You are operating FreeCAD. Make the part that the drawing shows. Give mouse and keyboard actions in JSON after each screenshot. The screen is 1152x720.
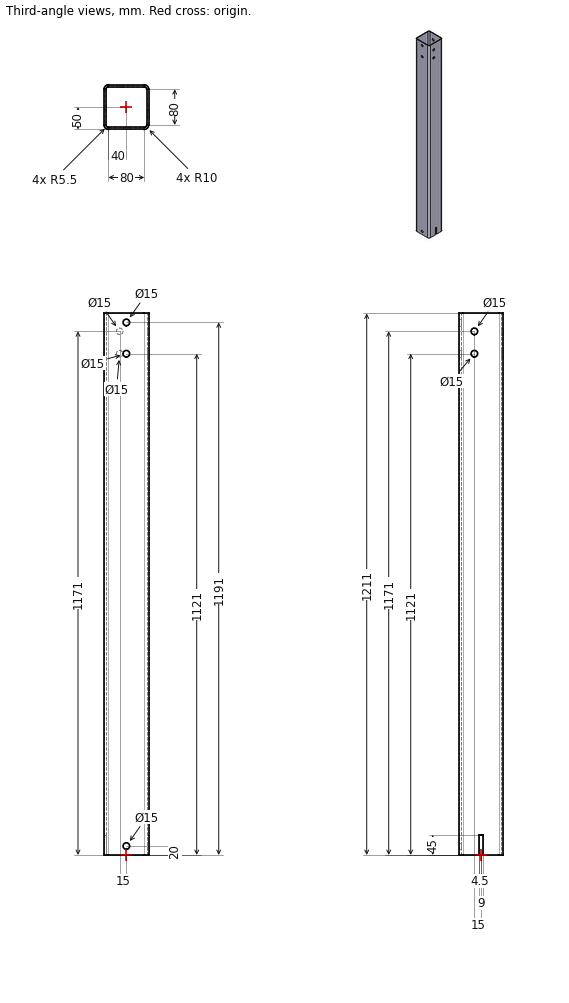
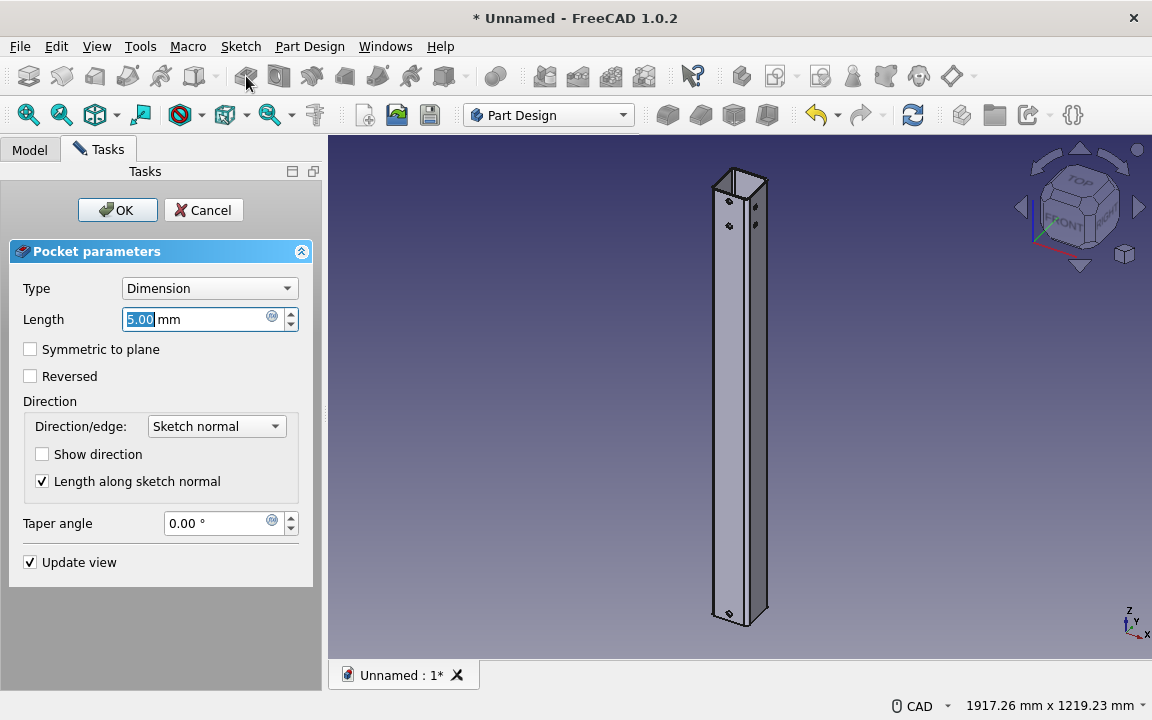
{"action": "left_click", "coordinate": [210, 288]}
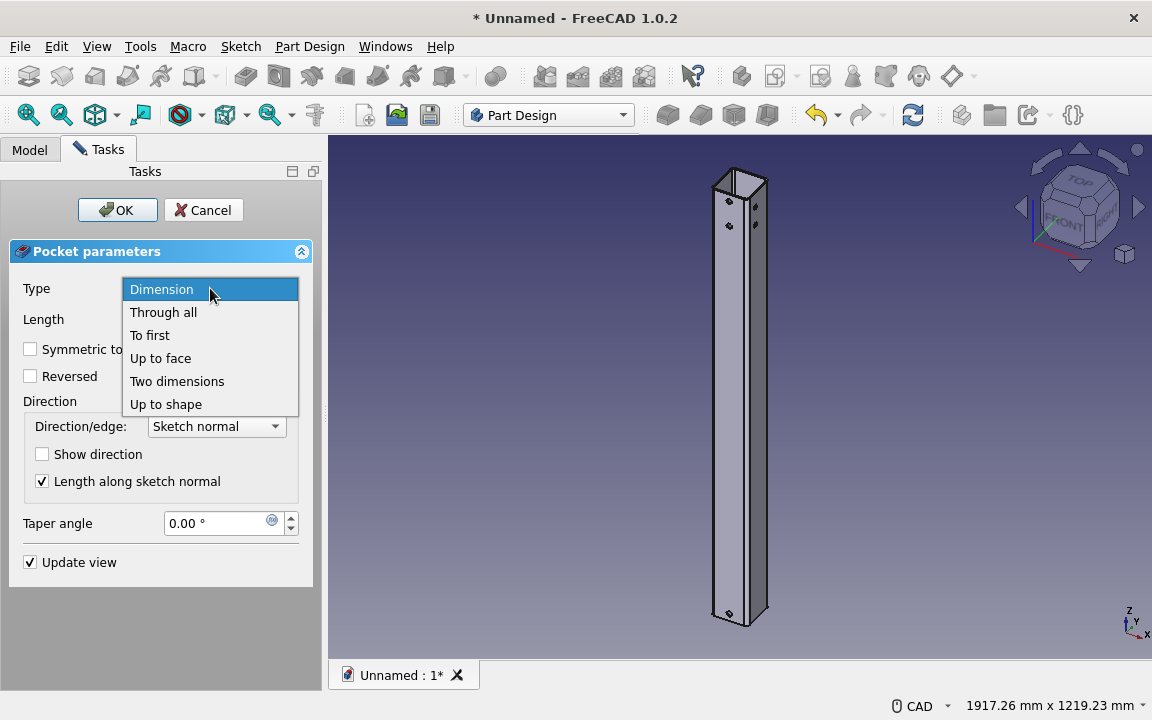
{"action": "left_click", "coordinate": [208, 336]}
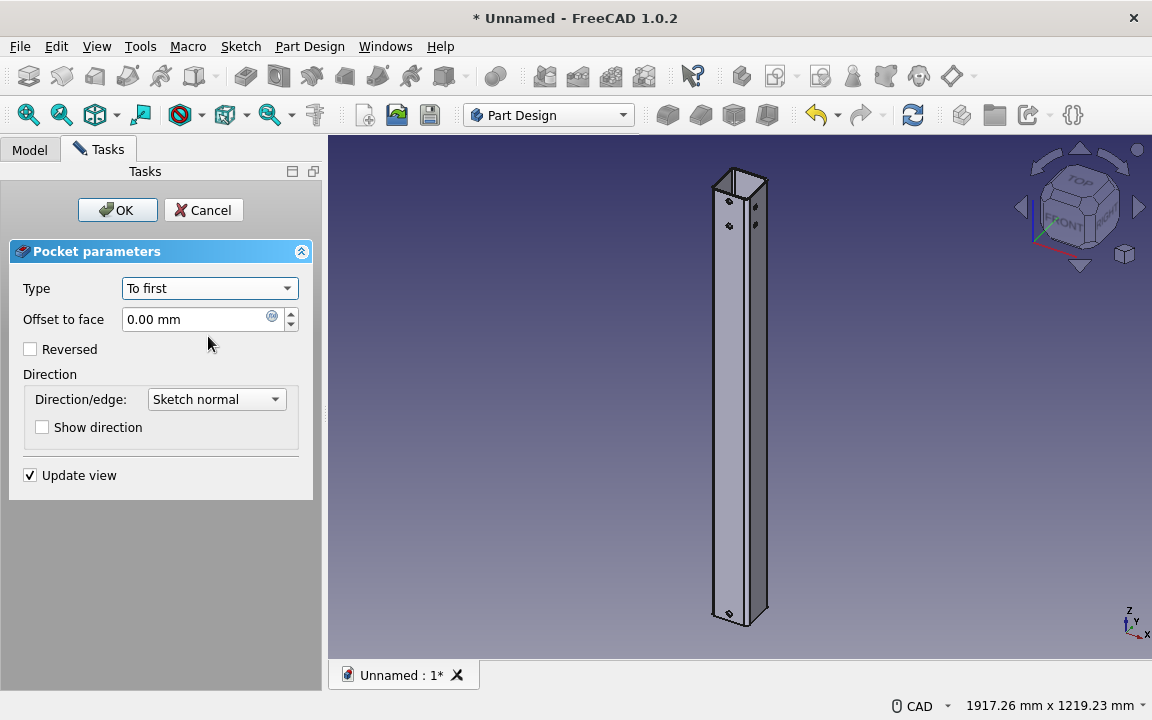
{"action": "left_click", "coordinate": [118, 210]}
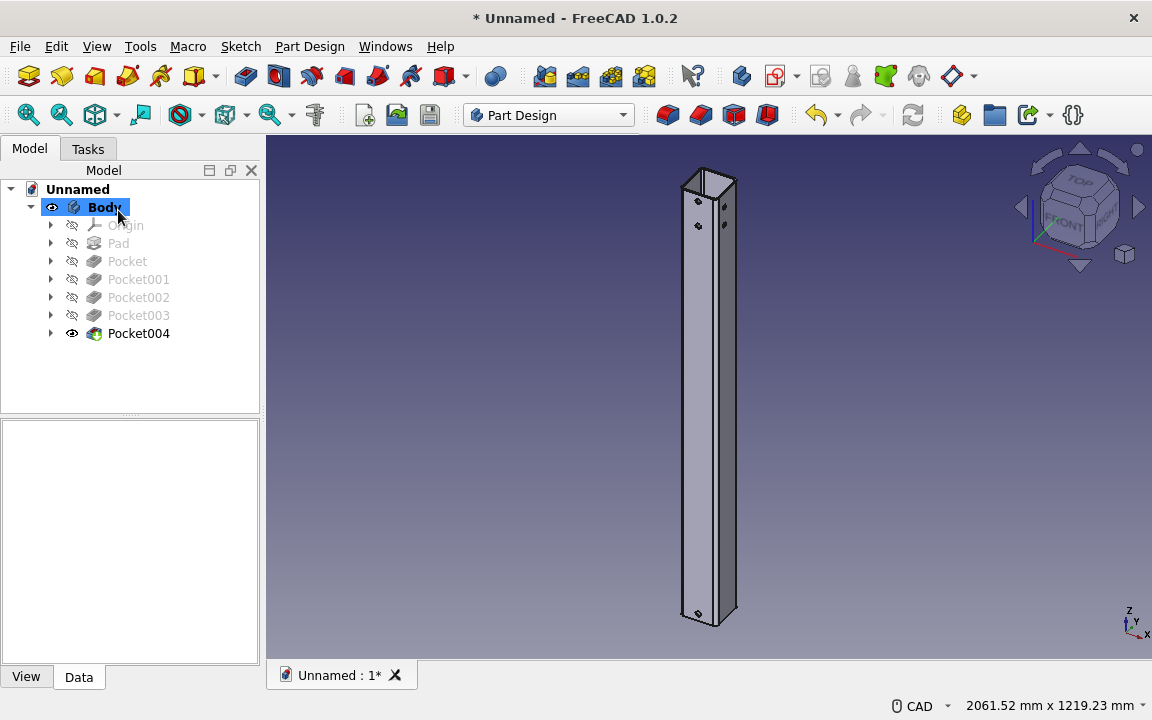
{"action": "key", "text": "4"}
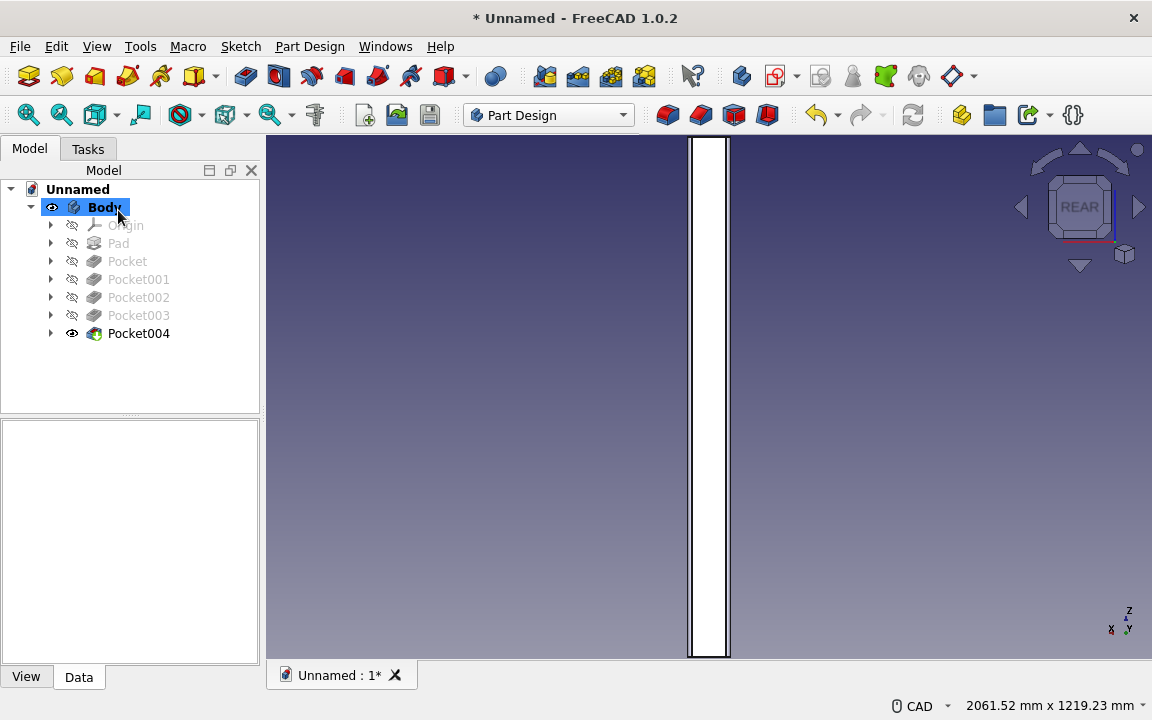
{"action": "left_click", "coordinate": [709, 173]}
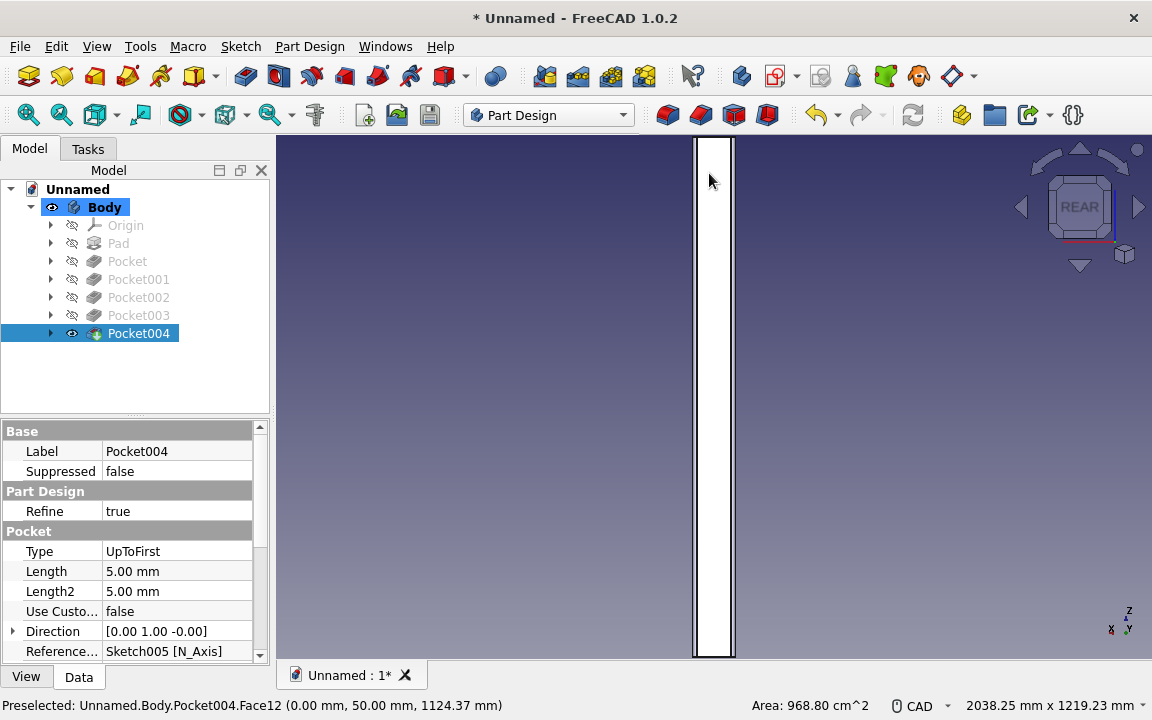
{"action": "left_click", "coordinate": [774, 76]}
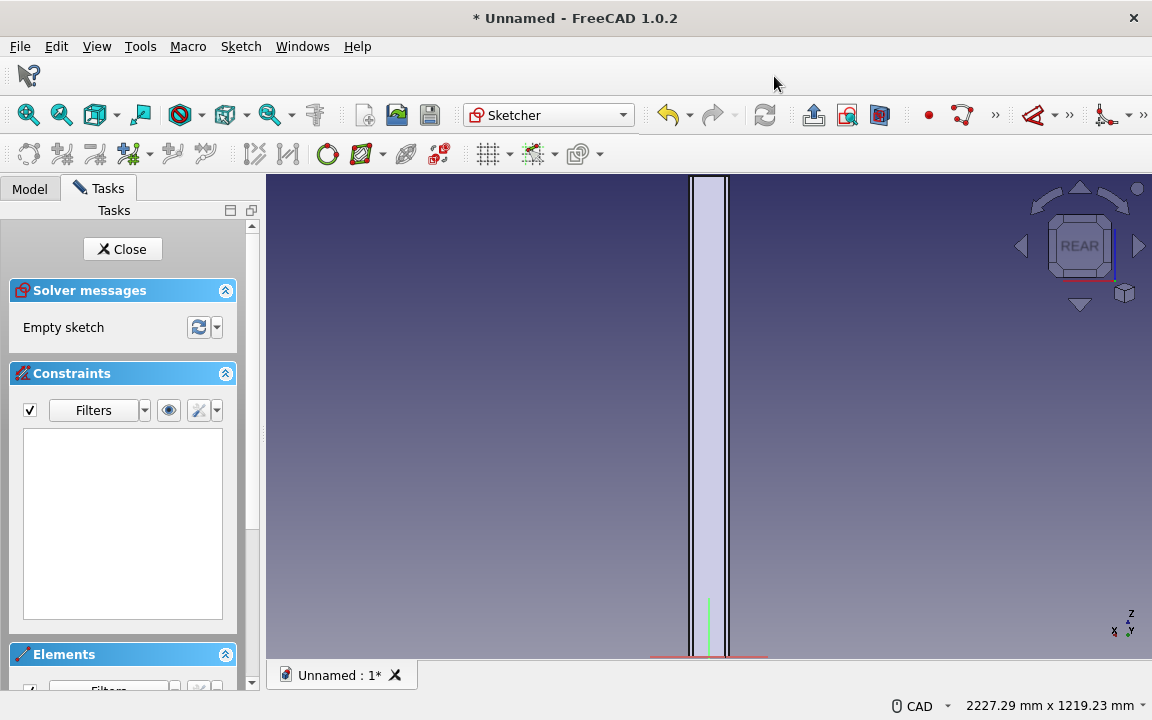
{"action": "scroll", "coordinate": [640, 416], "scroll_direction": "down", "scroll_amount": 5}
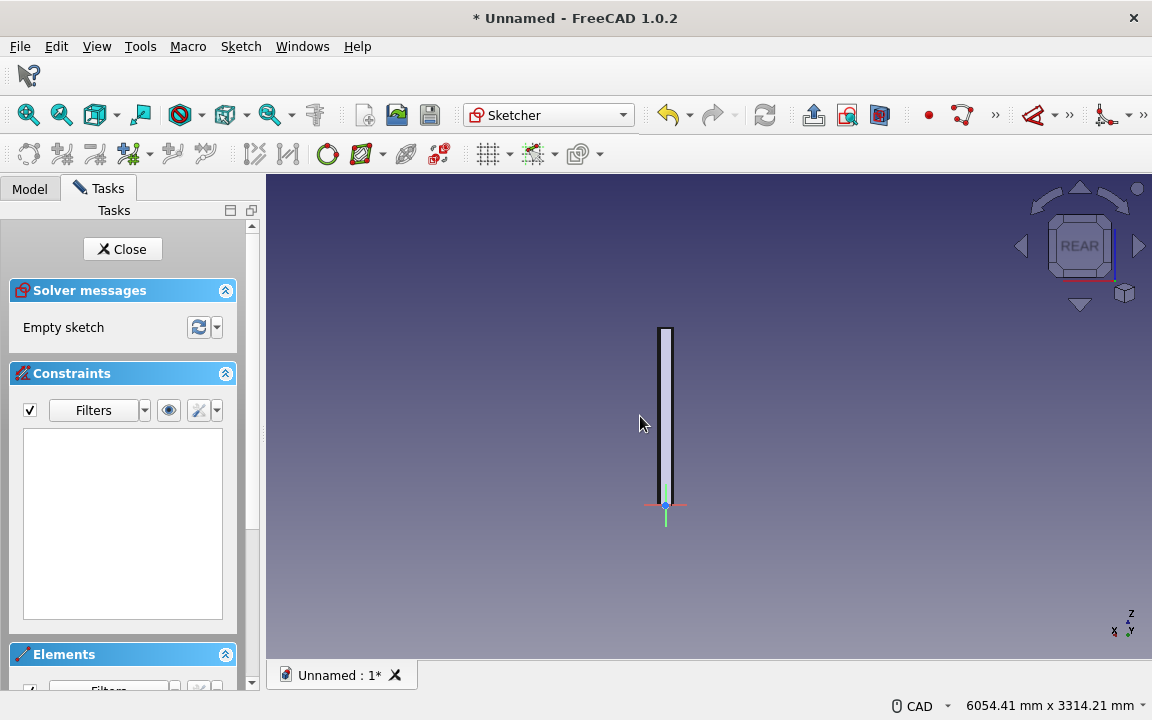
{"action": "scroll", "coordinate": [669, 329], "scroll_direction": "up", "scroll_amount": 15}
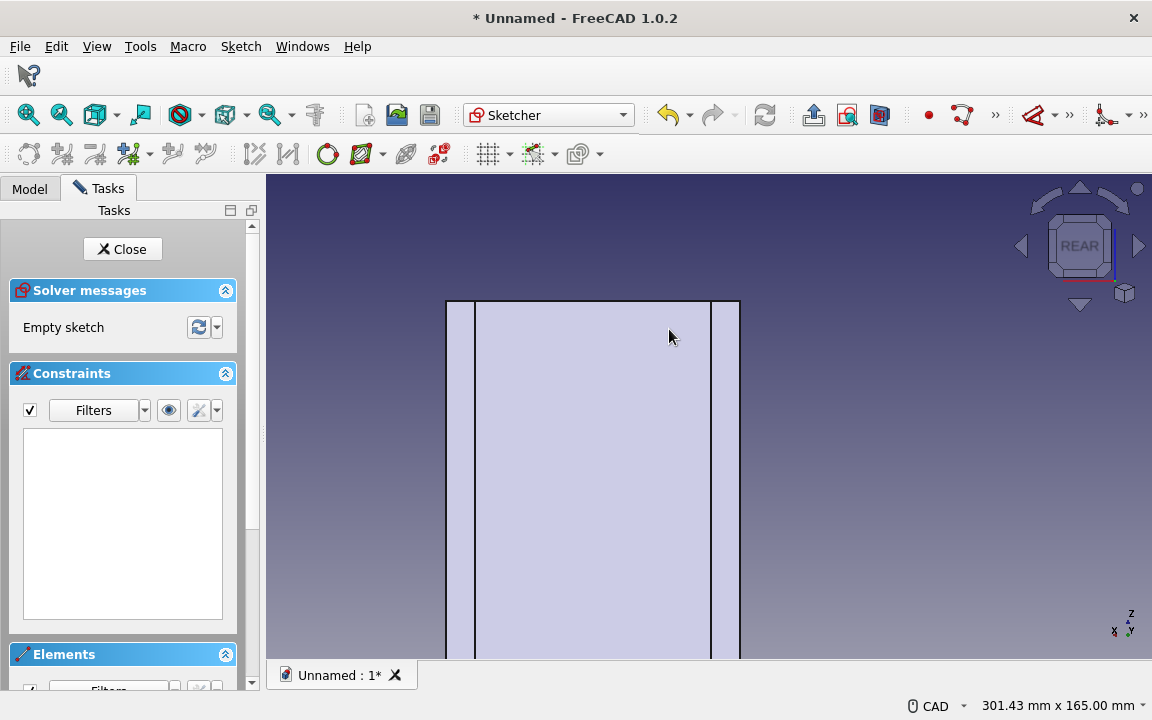
{"action": "scroll", "coordinate": [637, 418], "scroll_direction": "up", "scroll_amount": 10}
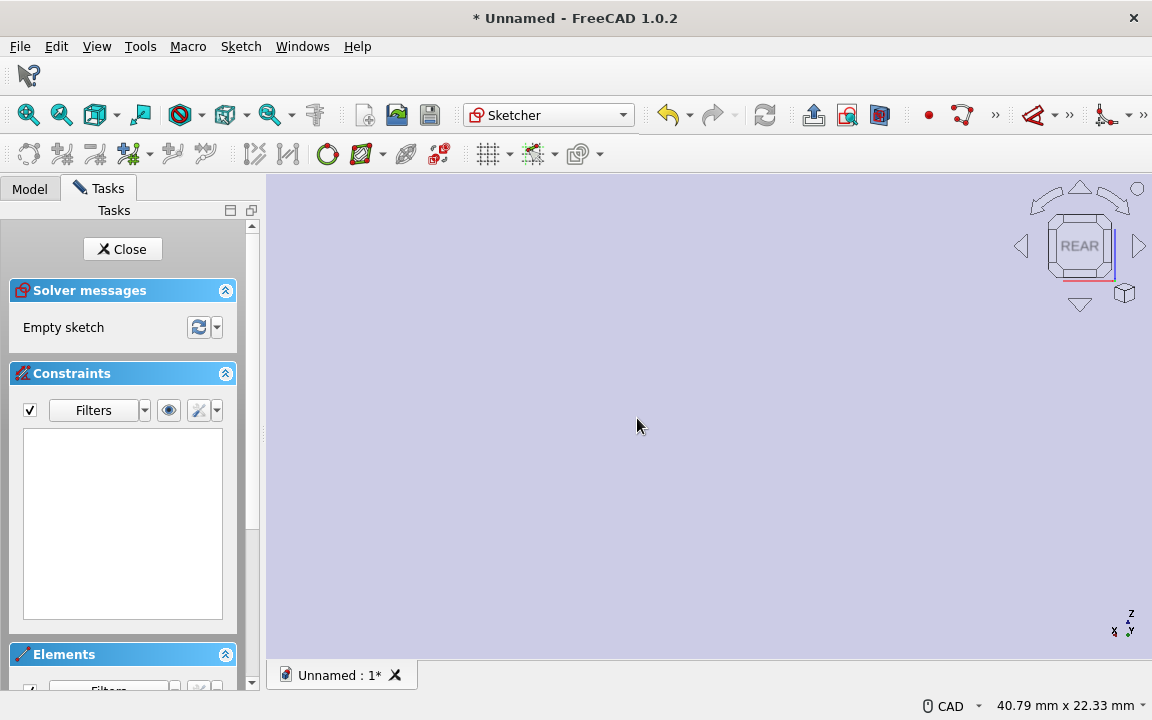
{"action": "key", "text": "g c"}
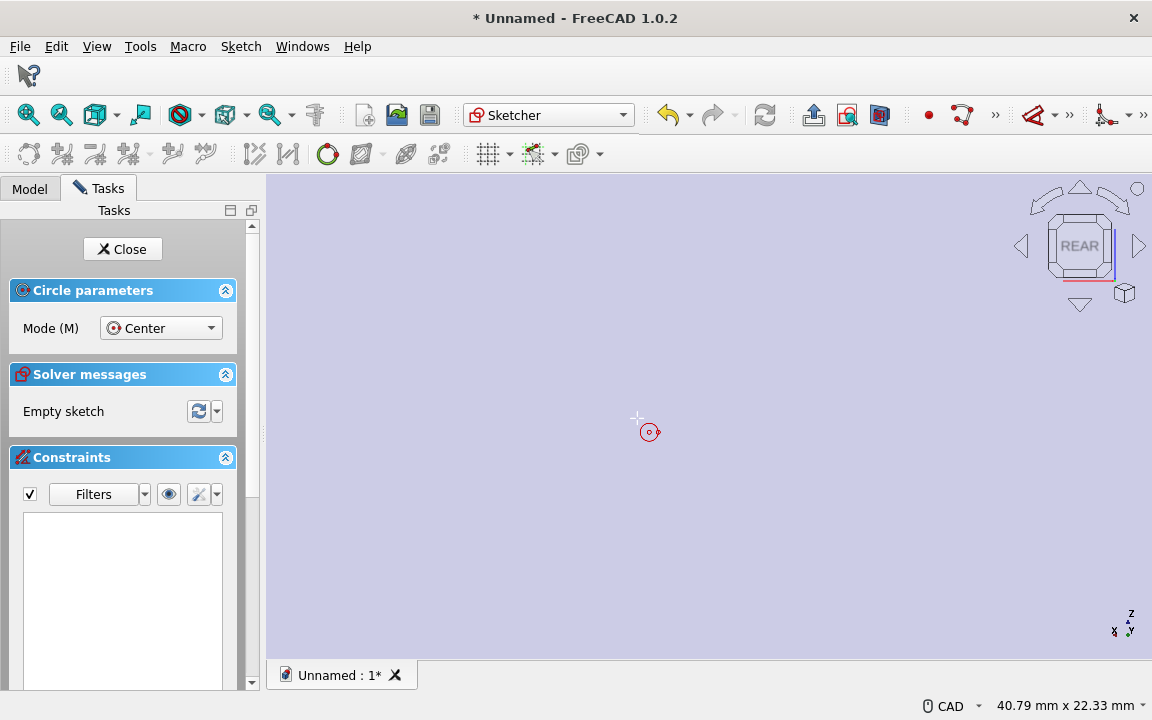
{"action": "left_click", "coordinate": [635, 416]}
{"action": "left_click", "coordinate": [750, 301]}
{"action": "key", "text": "Escape"}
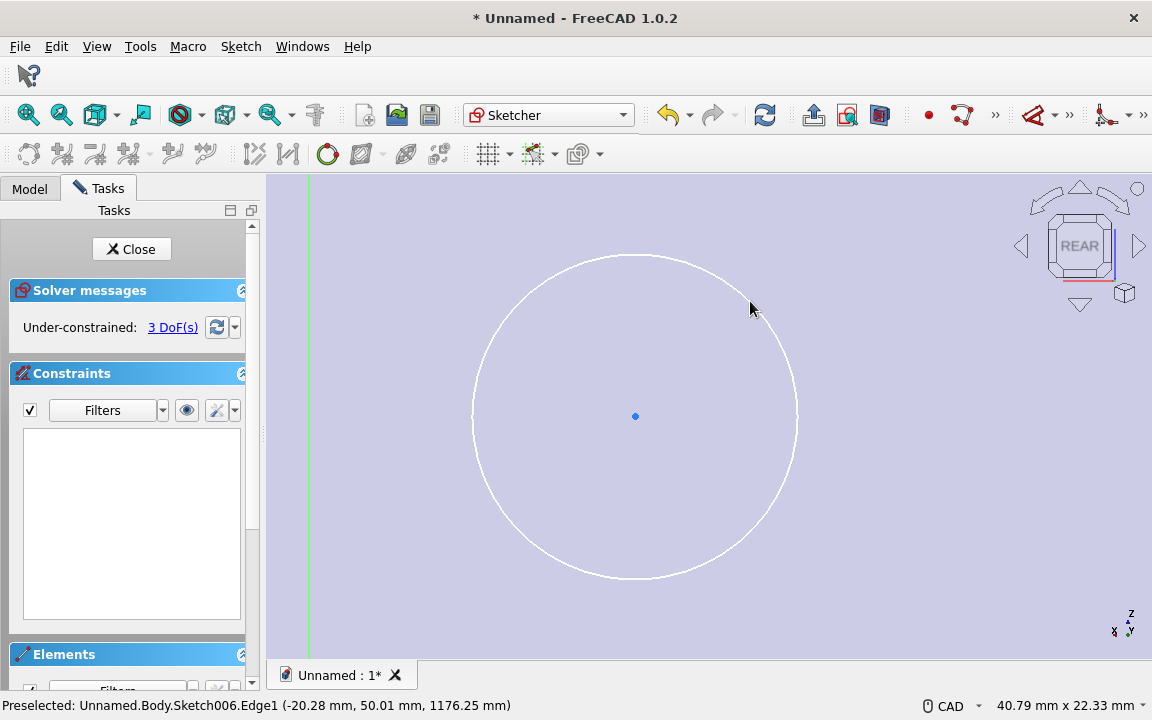
{"action": "left_click", "coordinate": [1032, 116]}